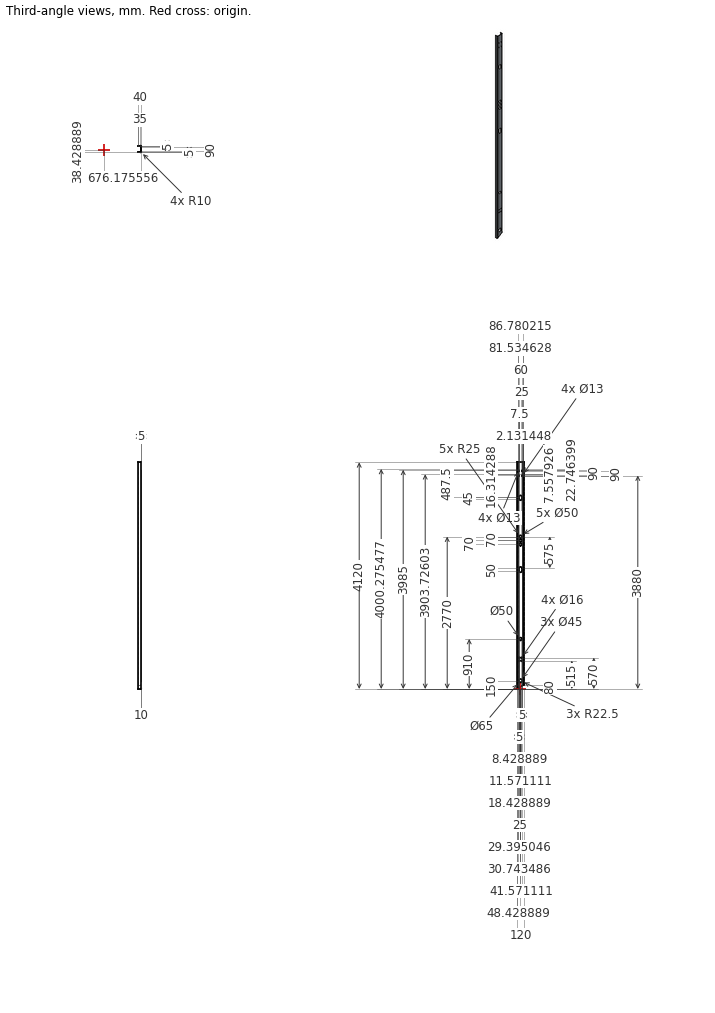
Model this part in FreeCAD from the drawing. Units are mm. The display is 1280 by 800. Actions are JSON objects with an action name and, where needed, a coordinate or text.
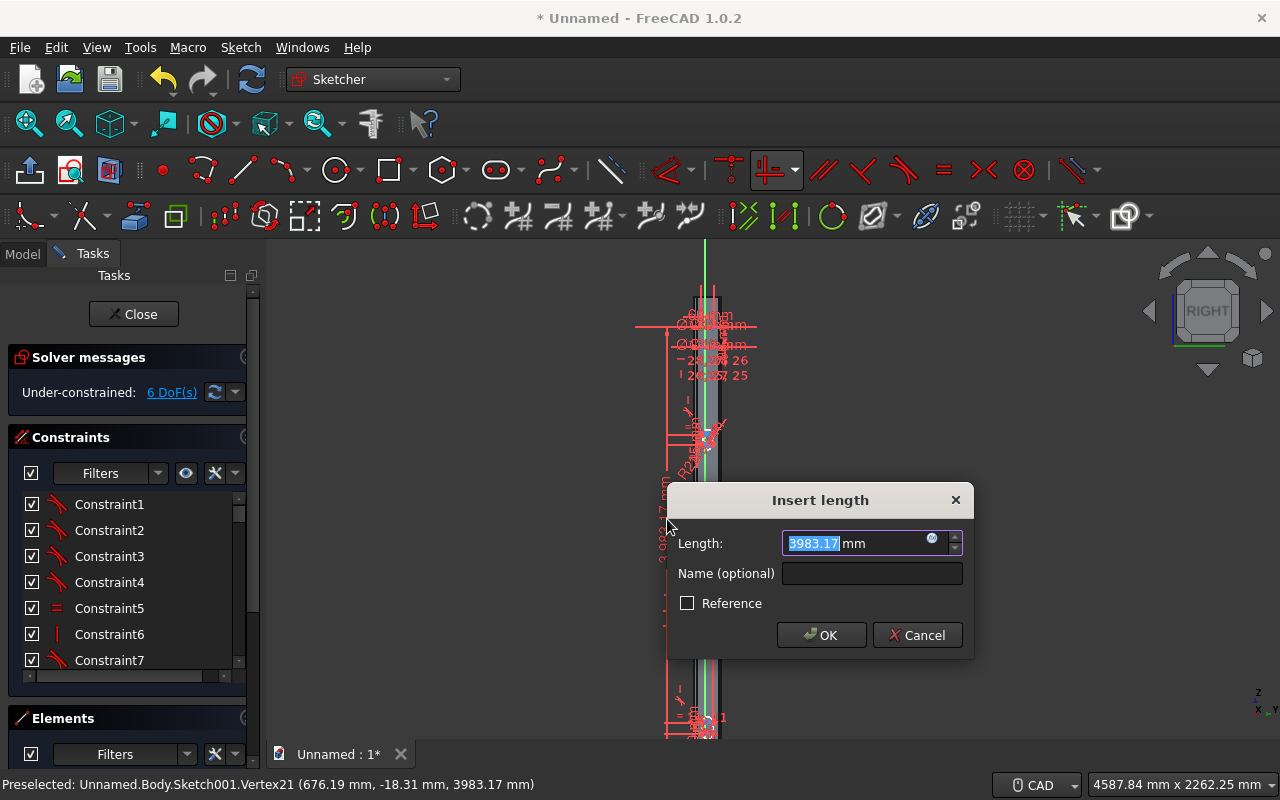
{"action": "type", "text": "3985"}
{"action": "key", "text": "Return"}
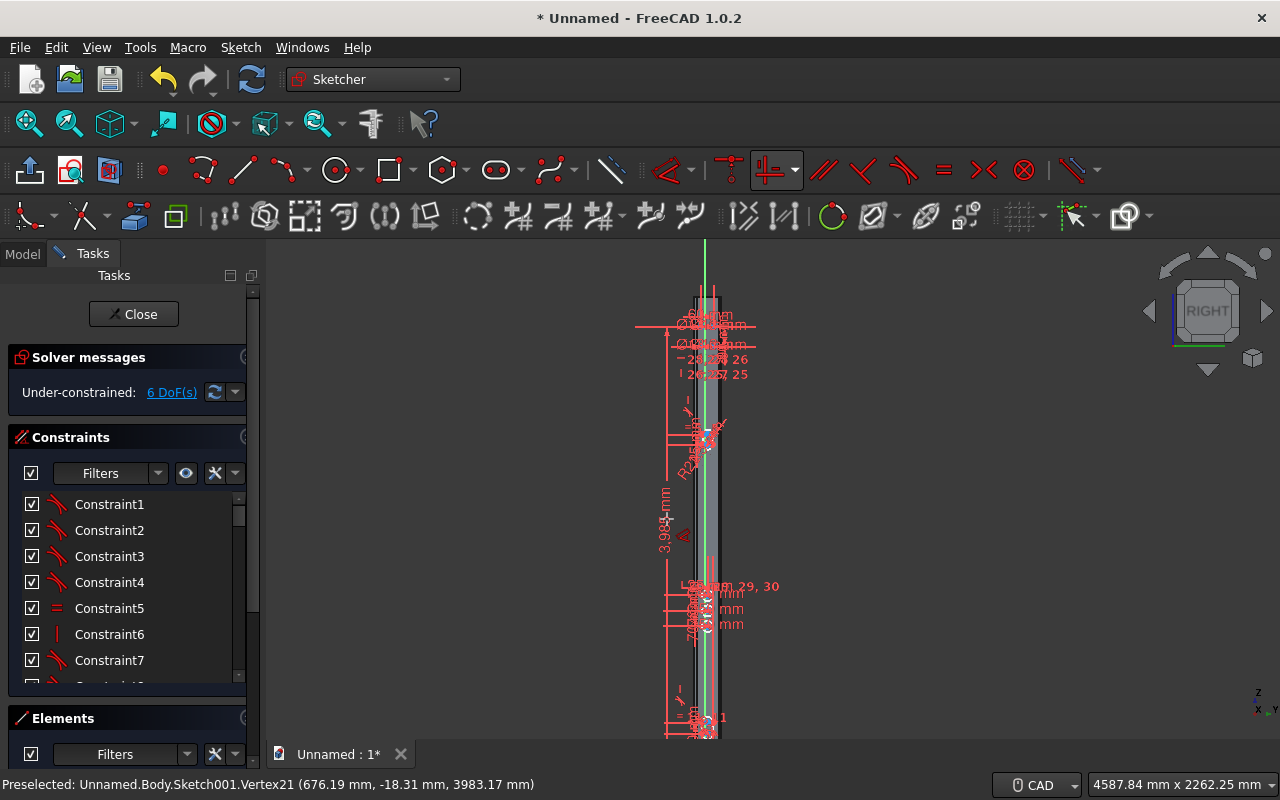
{"action": "left_click", "coordinate": [708, 595]}
{"action": "left_click", "coordinate": [671, 653]}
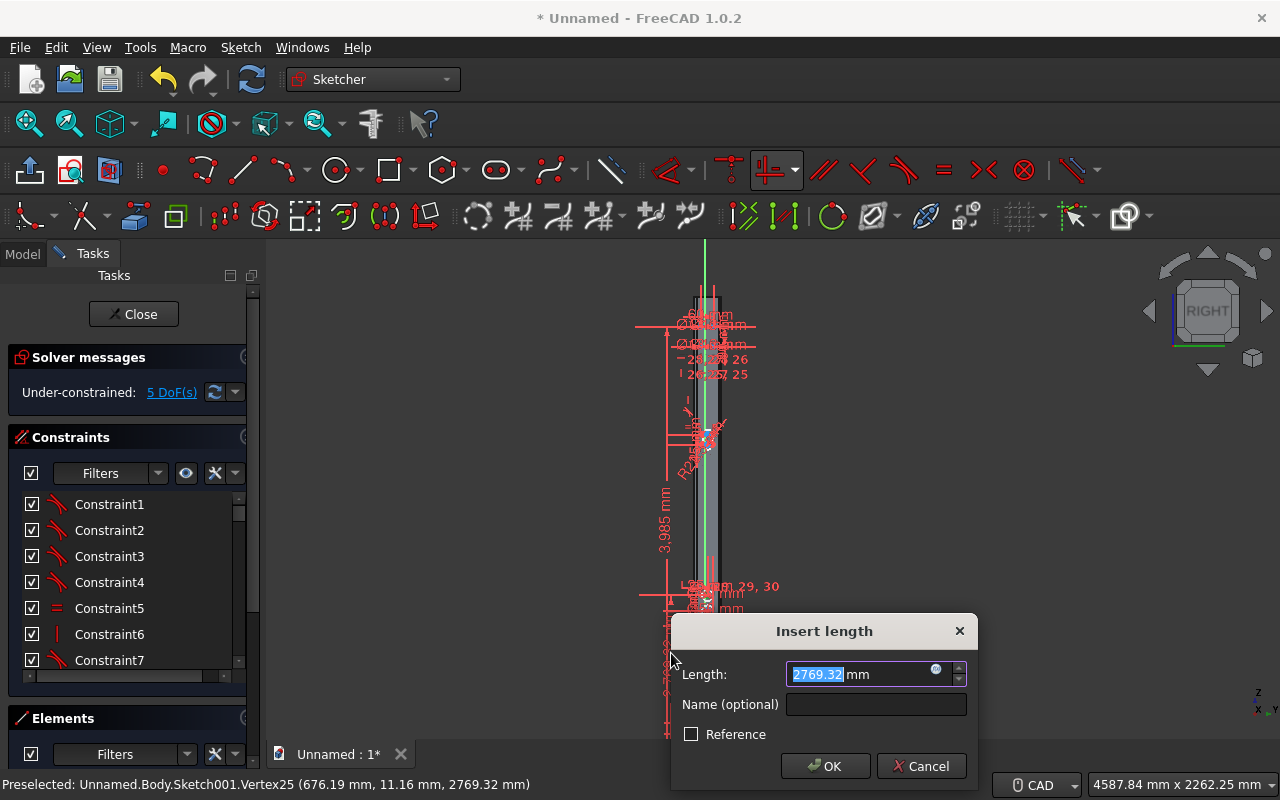
{"action": "type", "text": "2770"}
{"action": "key", "text": "Return"}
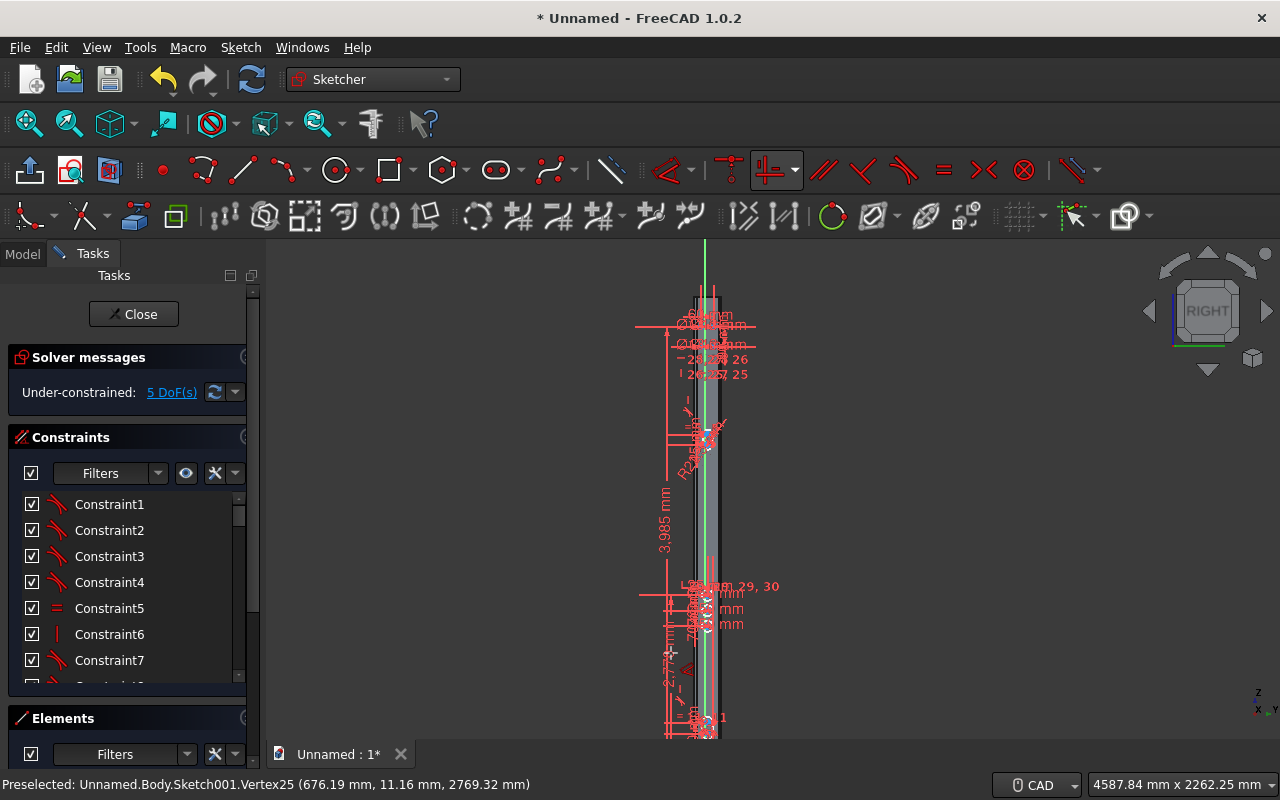
{"action": "scroll", "coordinate": [703, 435], "scroll_direction": "up", "scroll_amount": 16}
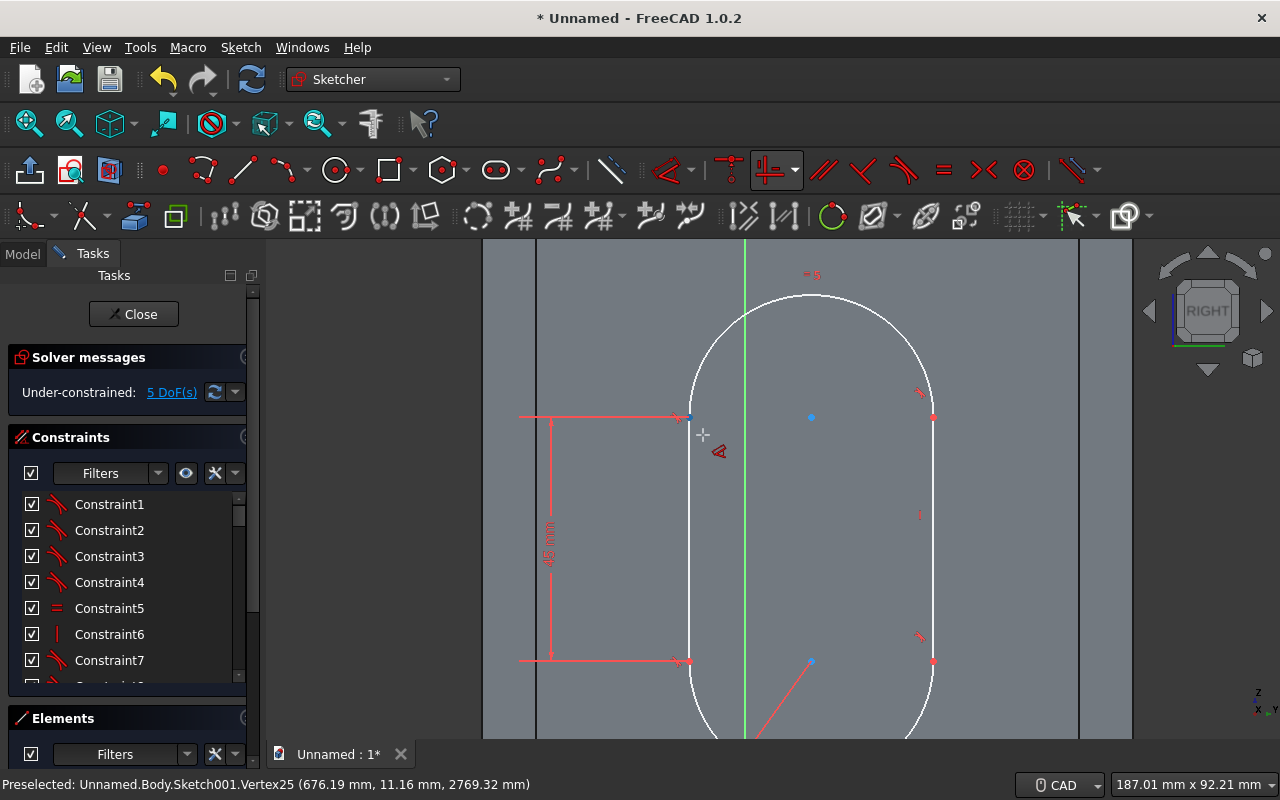
{"action": "left_click", "coordinate": [689, 417]}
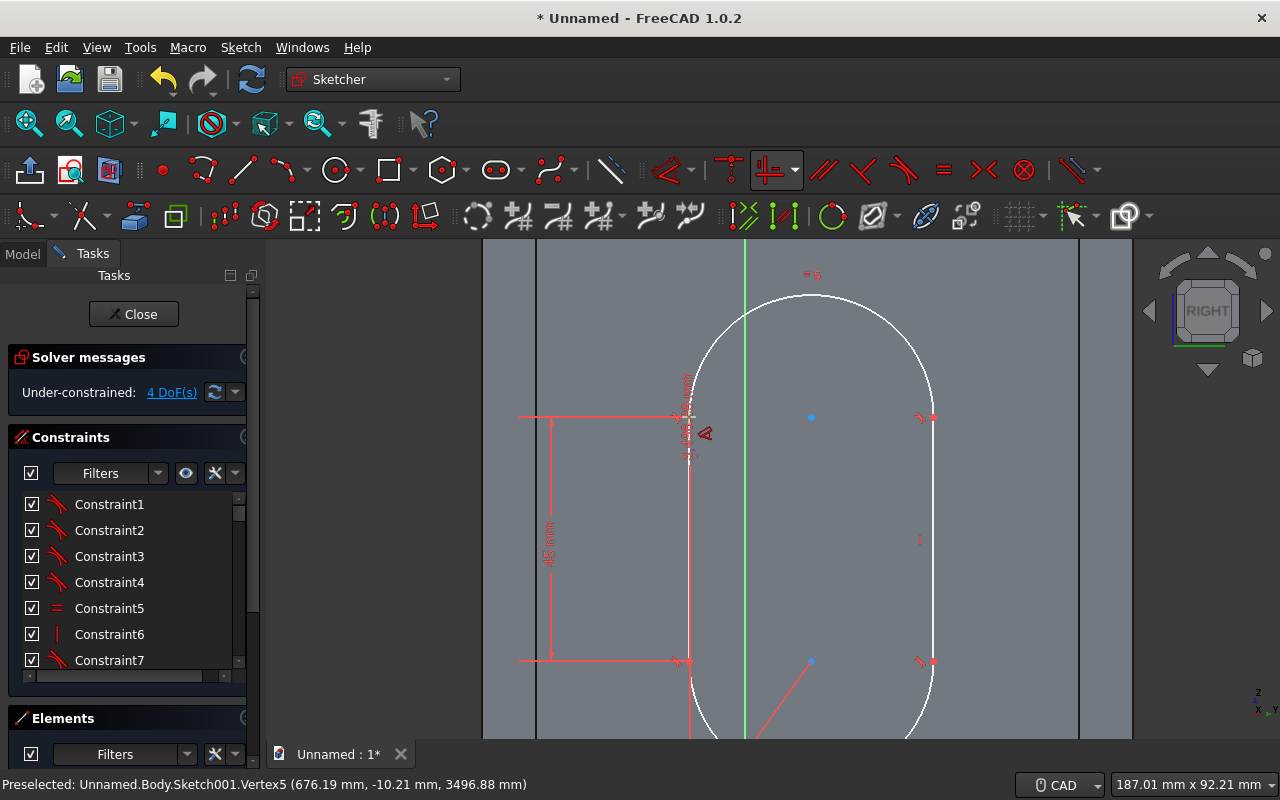
{"action": "scroll", "coordinate": [704, 489], "scroll_direction": "down", "scroll_amount": 15}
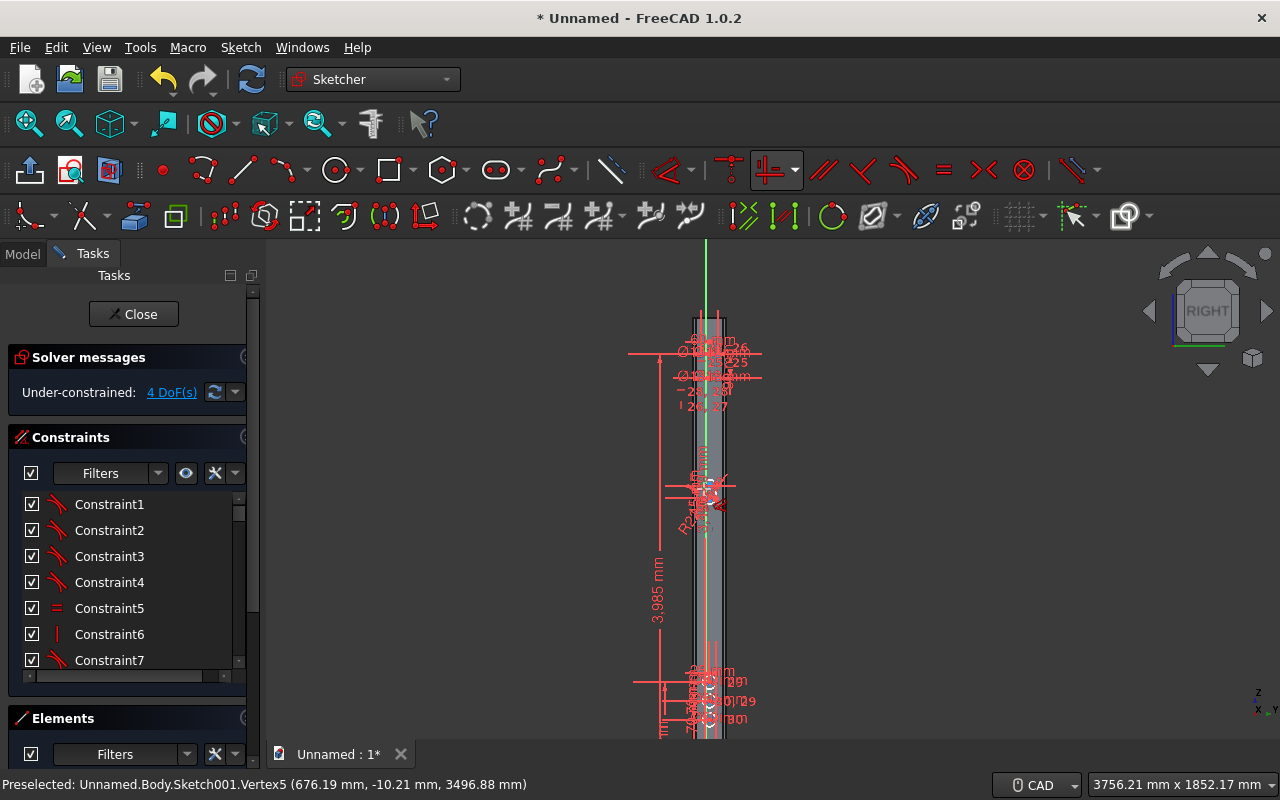
{"action": "scroll", "coordinate": [702, 316], "scroll_direction": "down", "scroll_amount": 6}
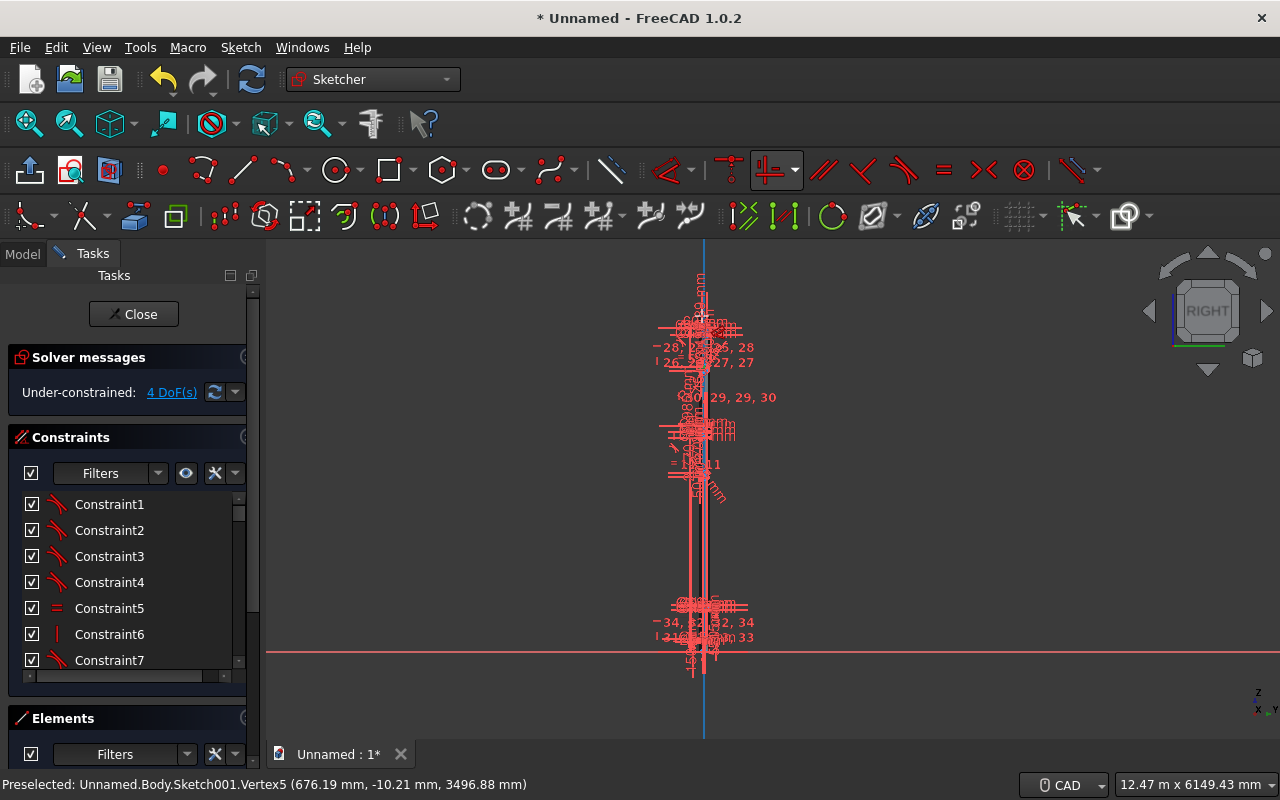
{"action": "scroll", "coordinate": [702, 328], "scroll_direction": "up", "scroll_amount": 21}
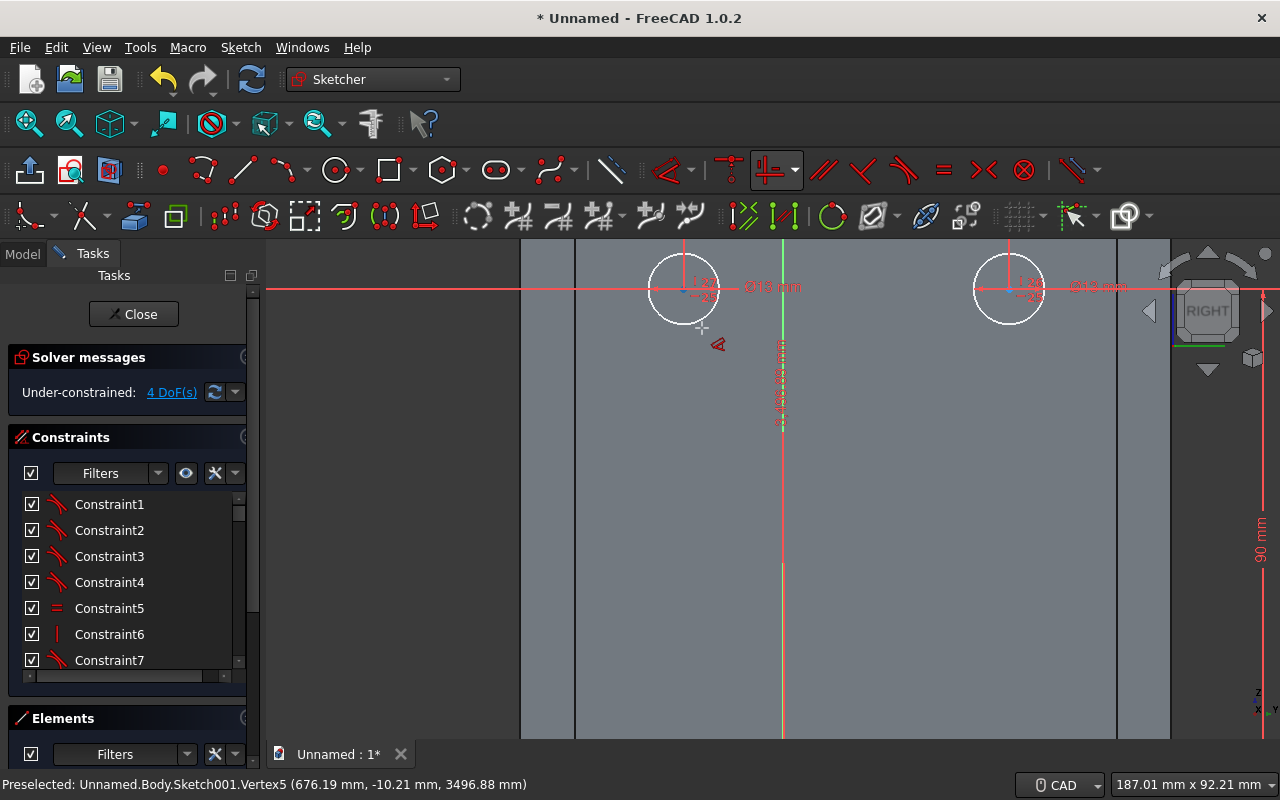
{"action": "left_click", "coordinate": [684, 289]}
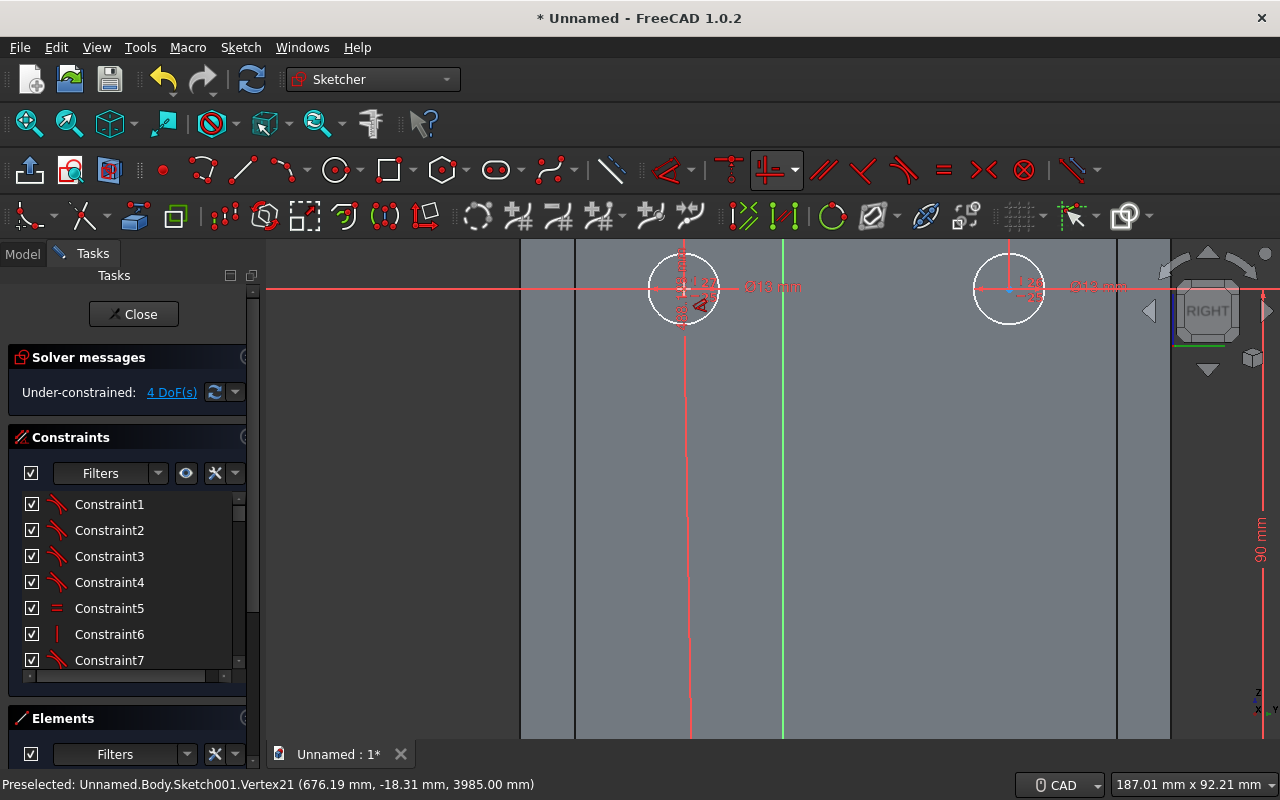
{"action": "key", "text": "Escape"}
{"action": "key", "text": "Escape"}